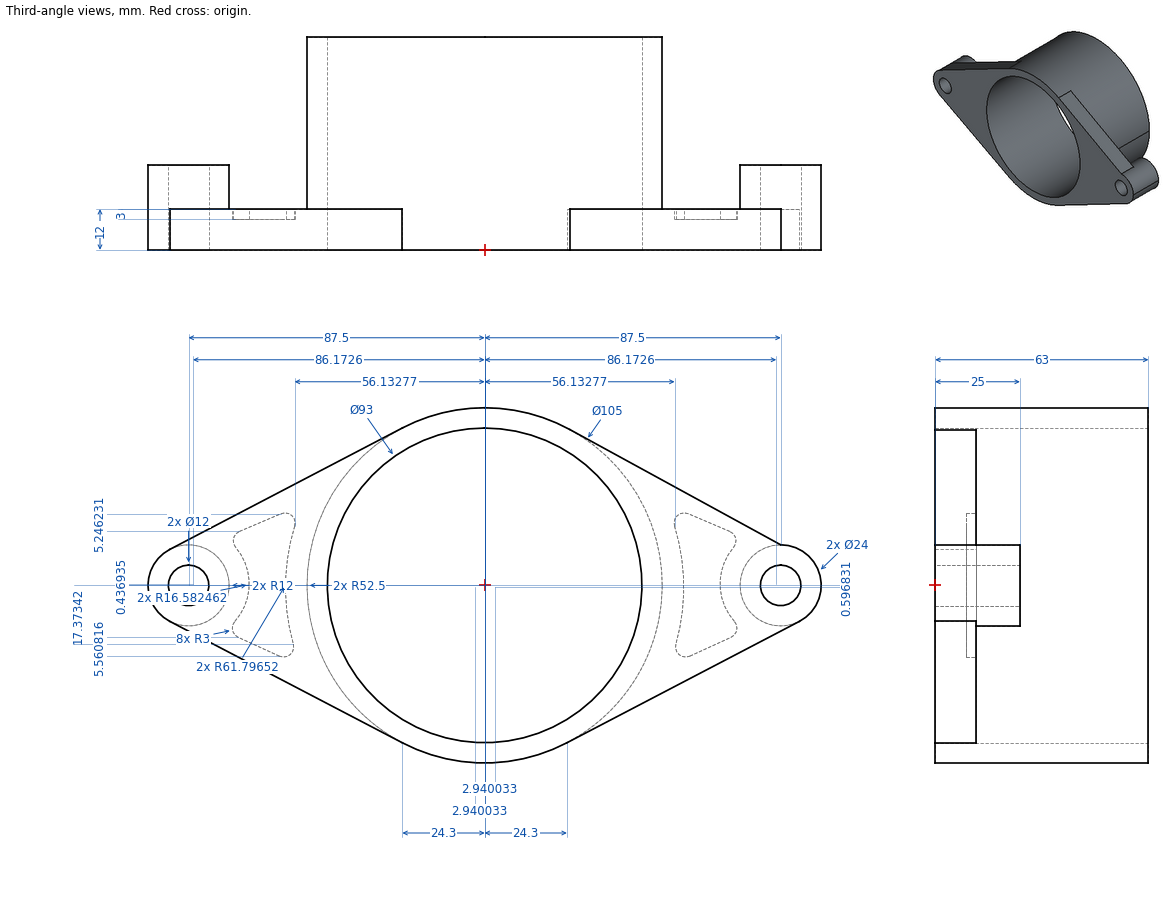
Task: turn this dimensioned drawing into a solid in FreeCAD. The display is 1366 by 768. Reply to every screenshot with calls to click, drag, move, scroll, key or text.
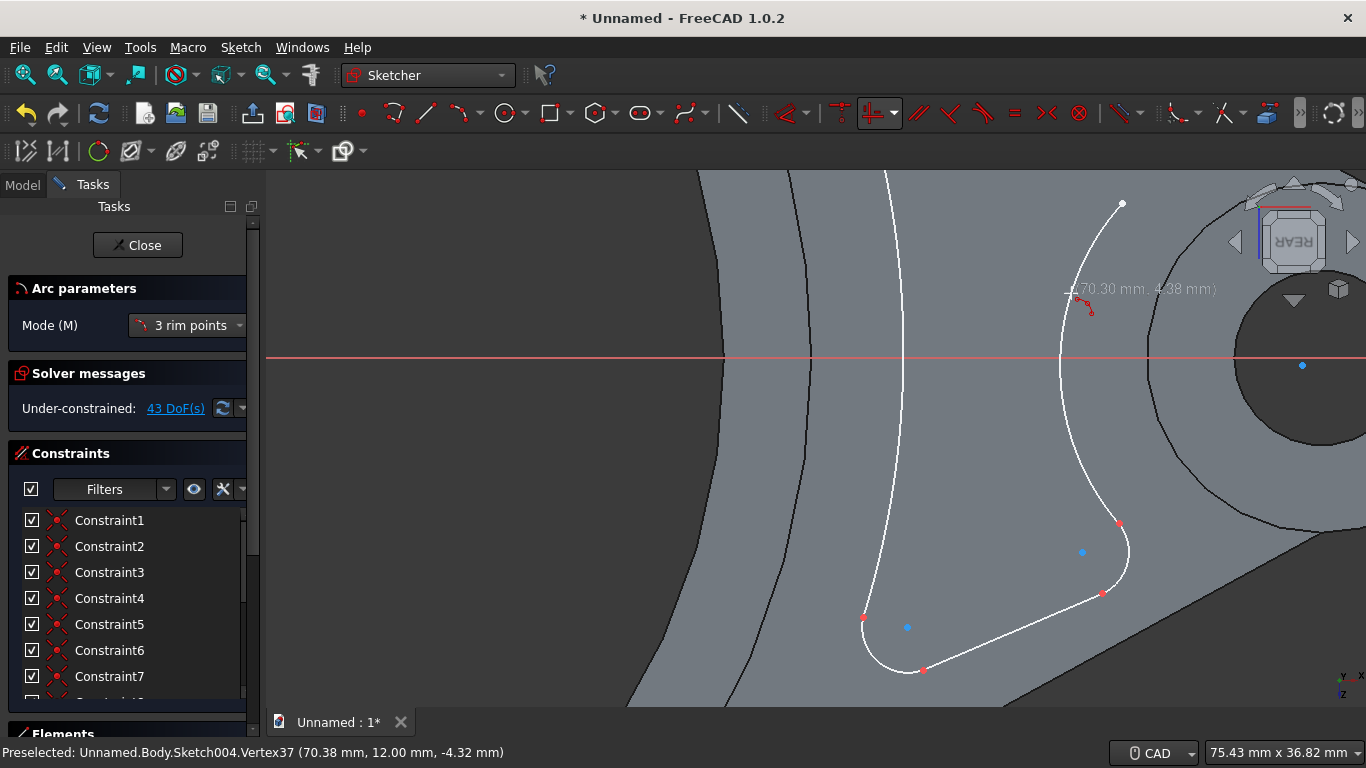
click(1122, 204)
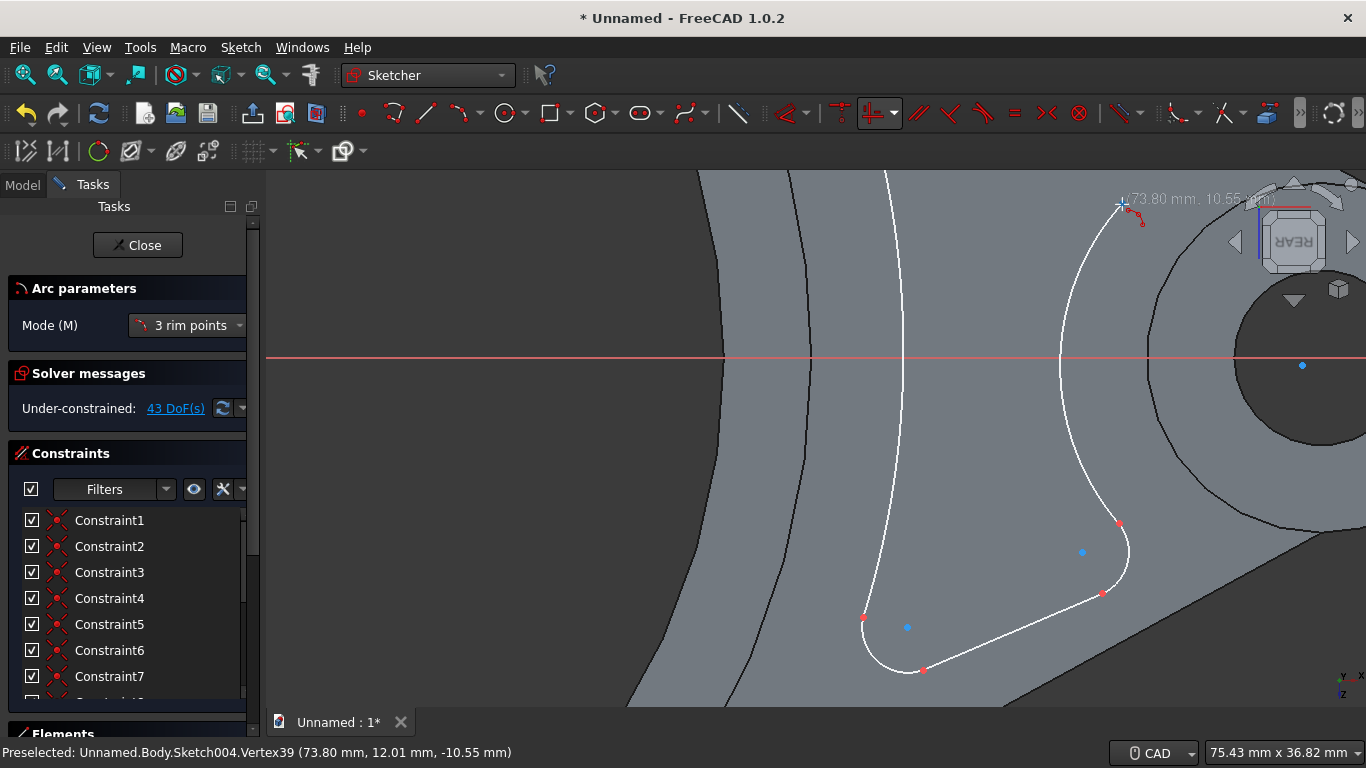
scroll(1050, 472, down, 6)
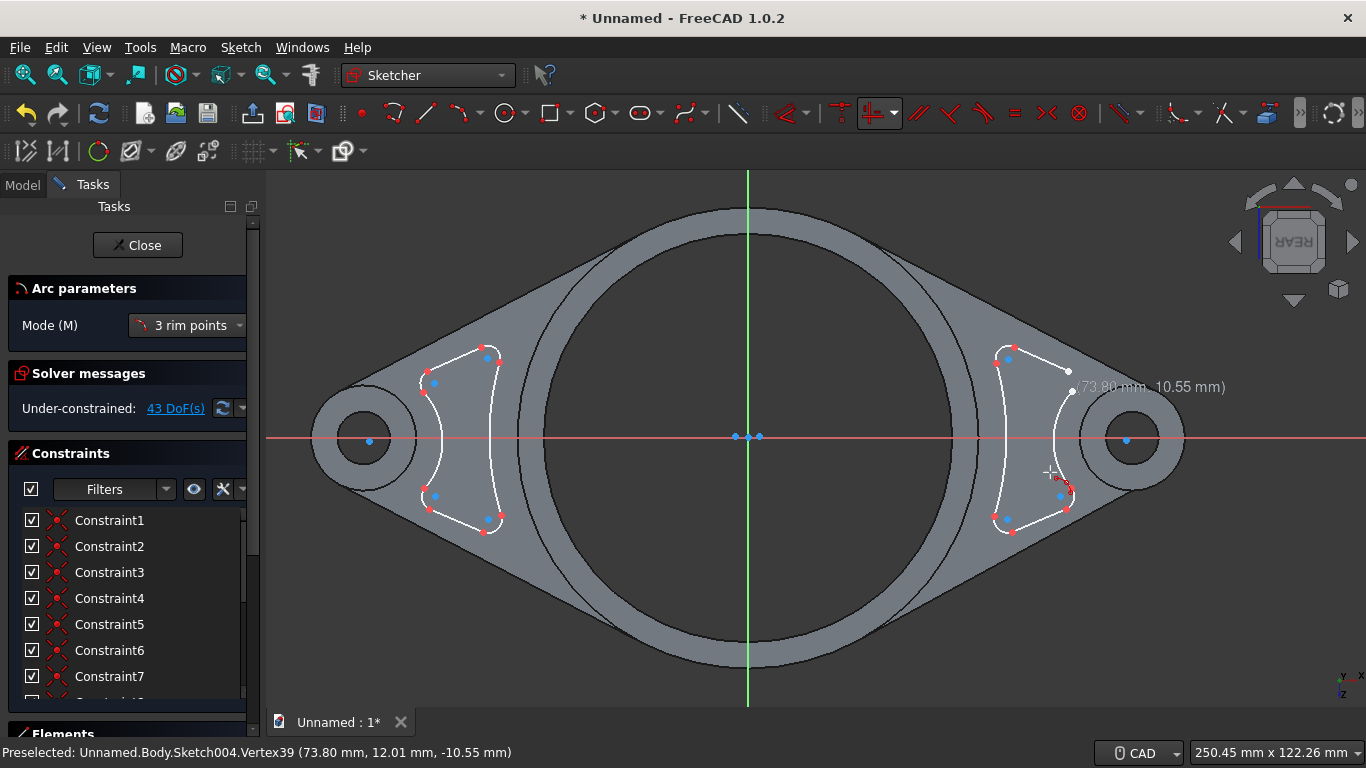
click(1068, 371)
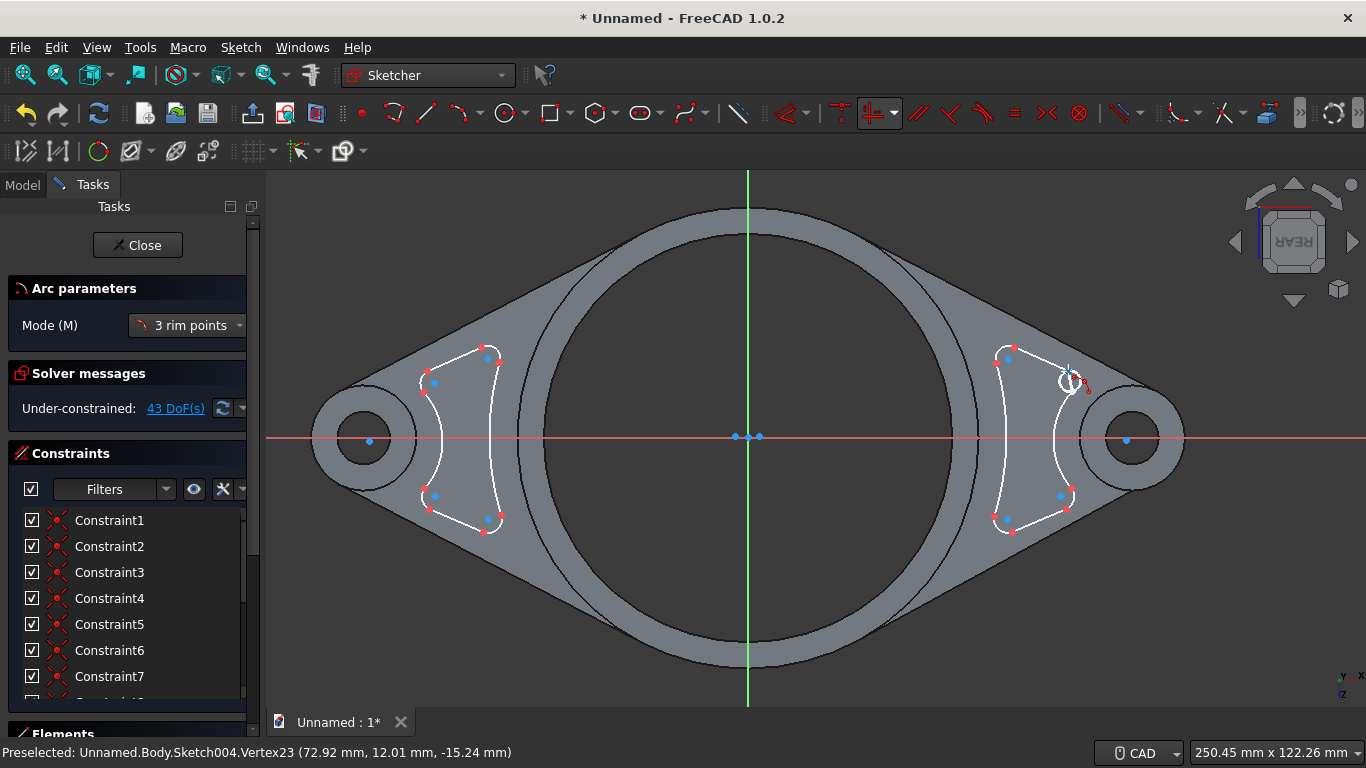
scroll(1075, 380, up, 6)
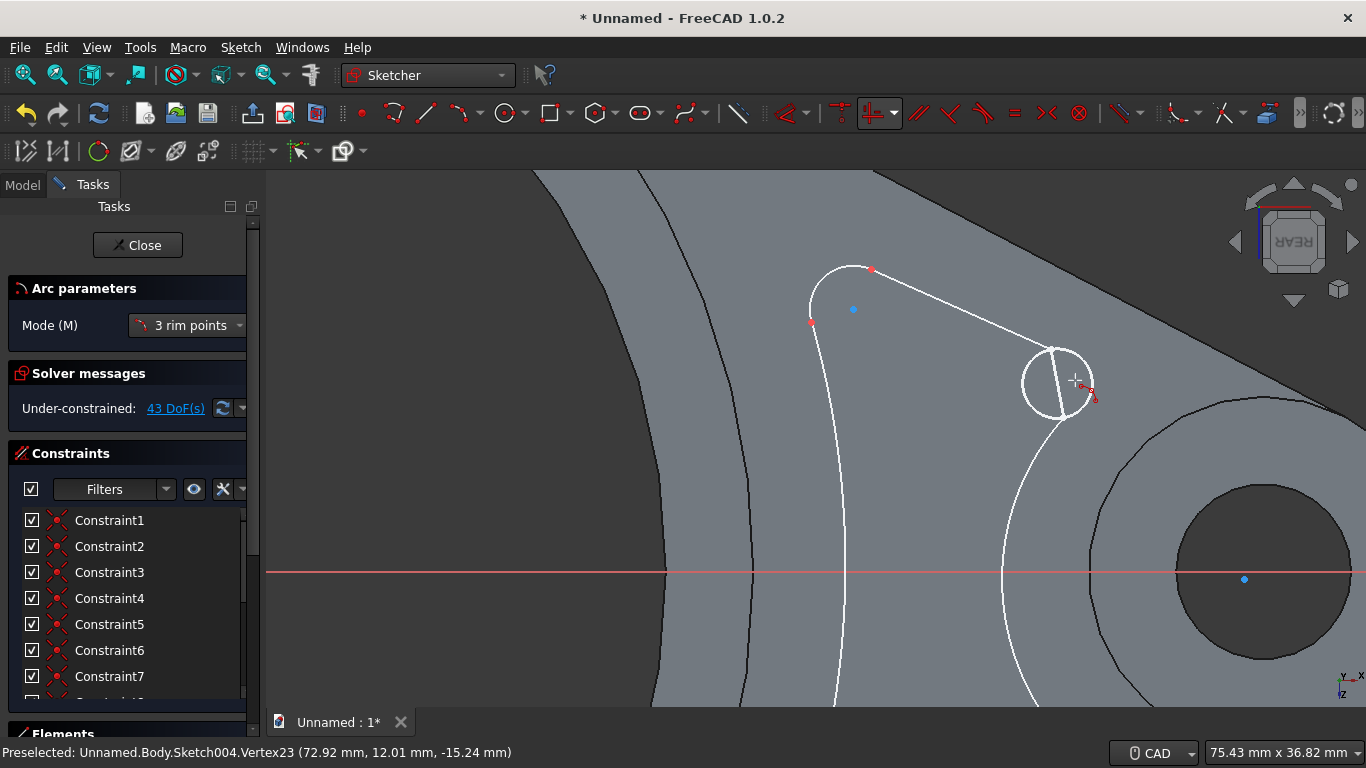
click(1074, 379)
key(Escape)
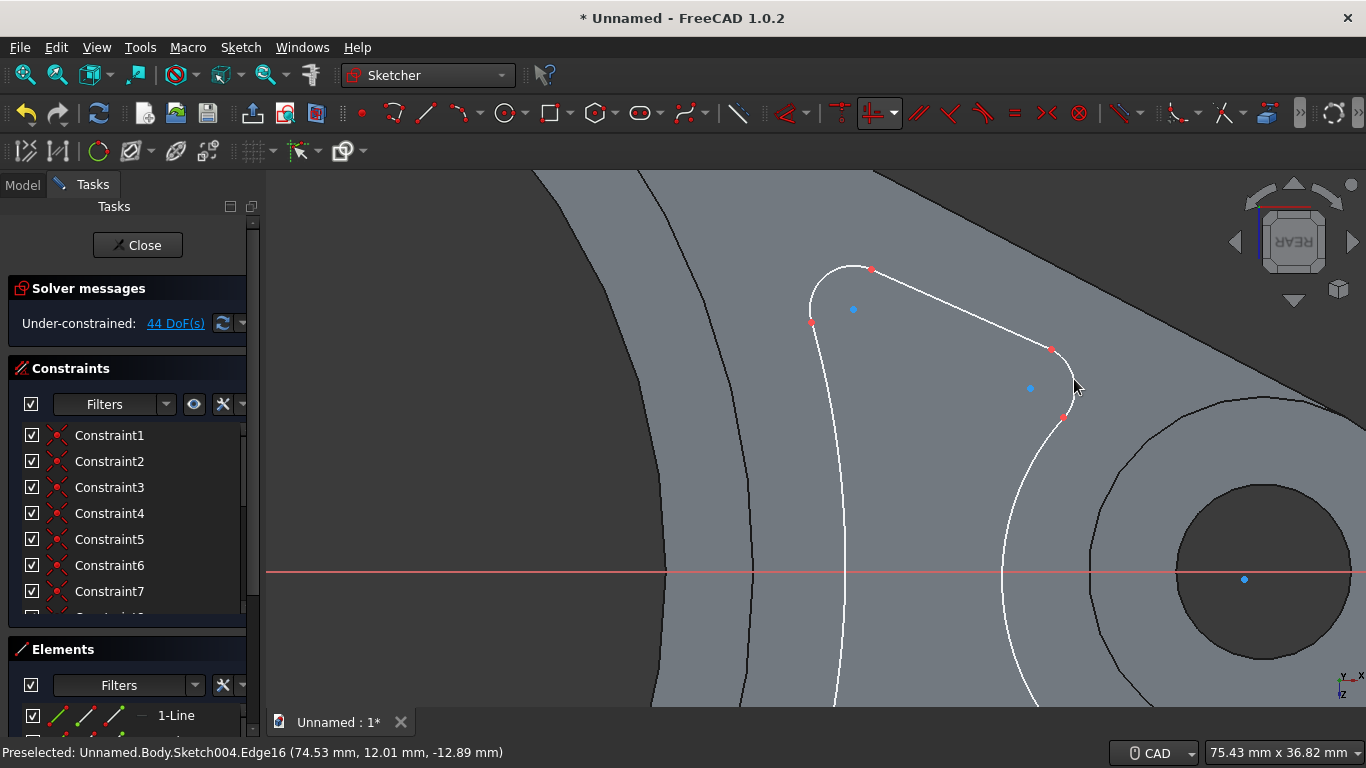
scroll(1075, 380, down, 6)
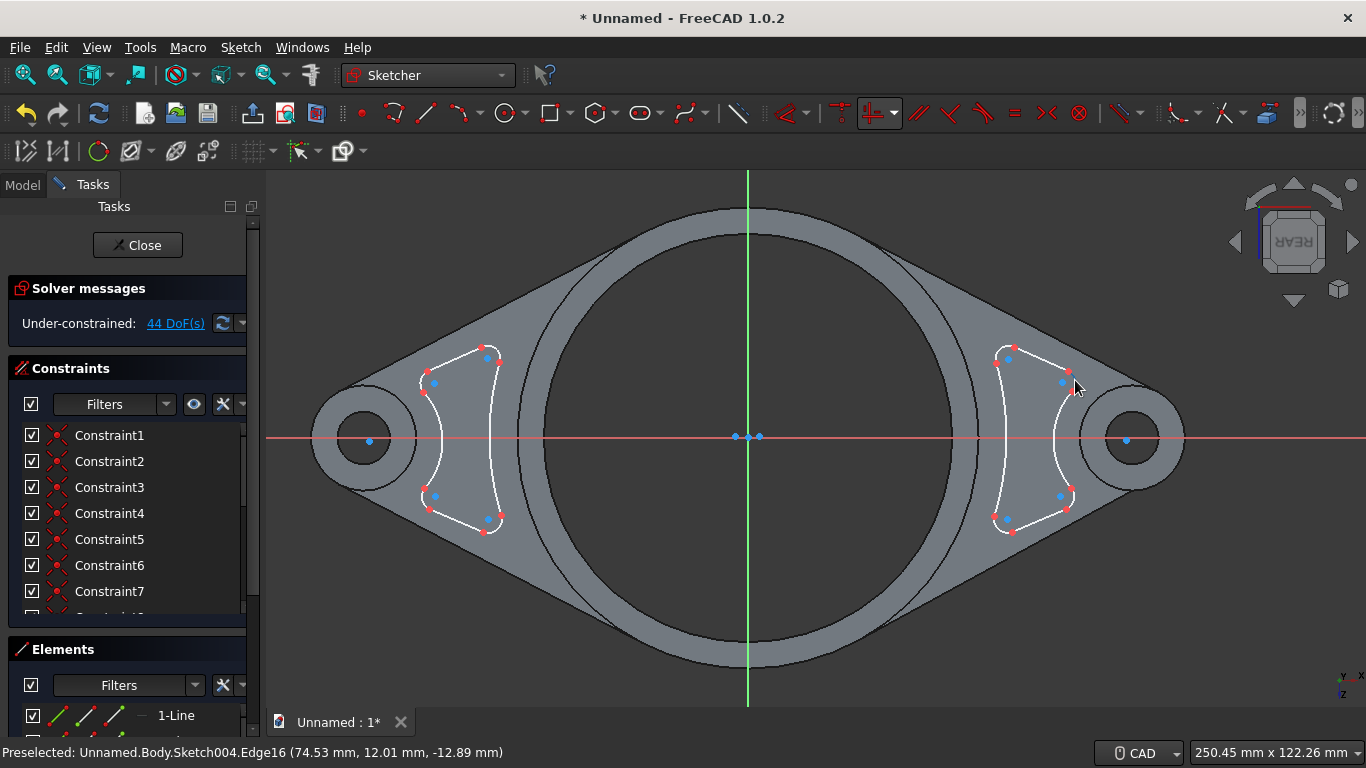
click(466, 355)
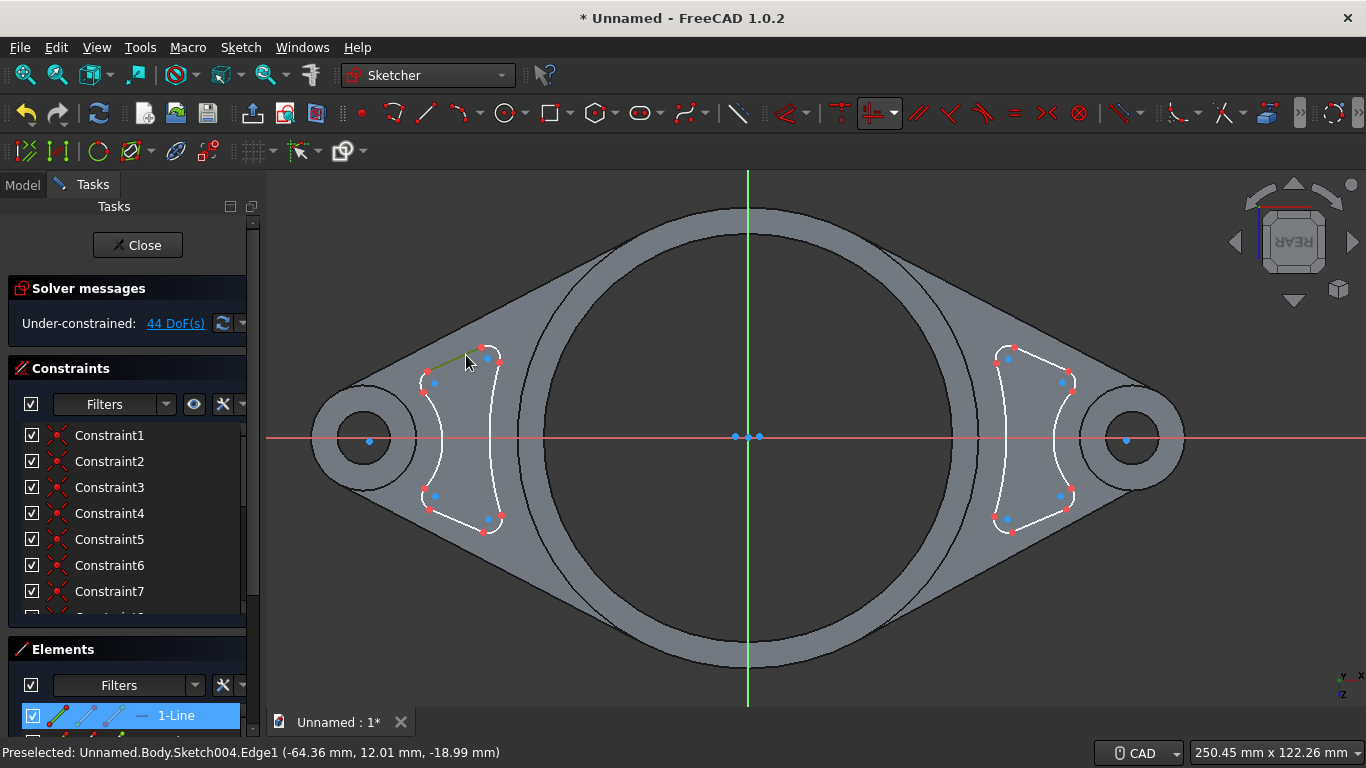
click(421, 381)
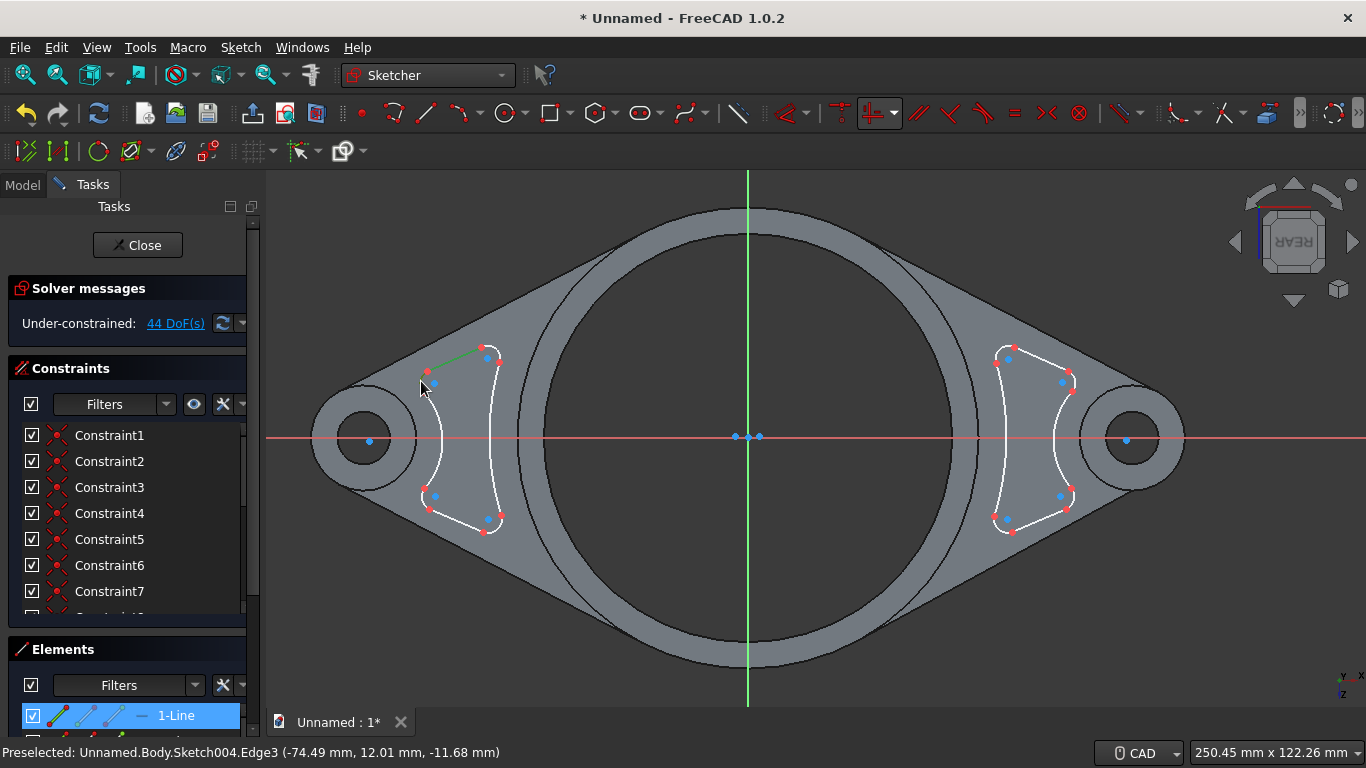
click(984, 114)